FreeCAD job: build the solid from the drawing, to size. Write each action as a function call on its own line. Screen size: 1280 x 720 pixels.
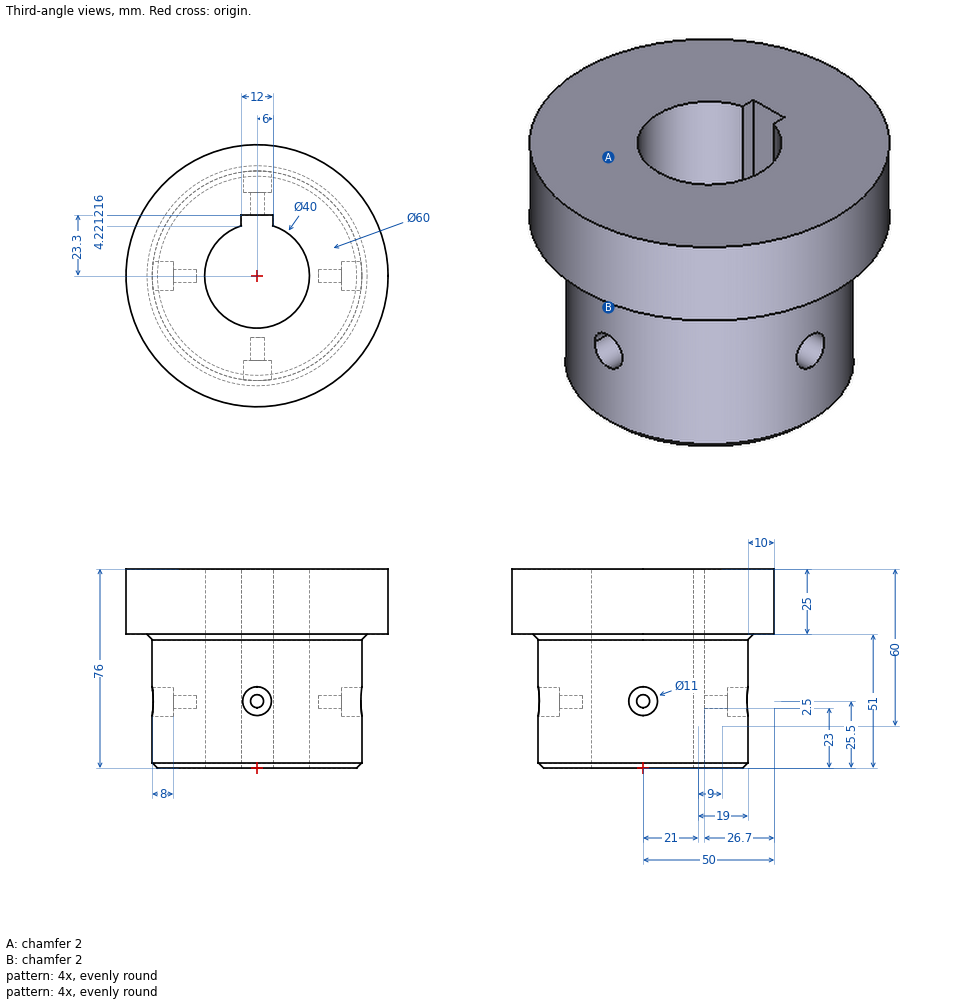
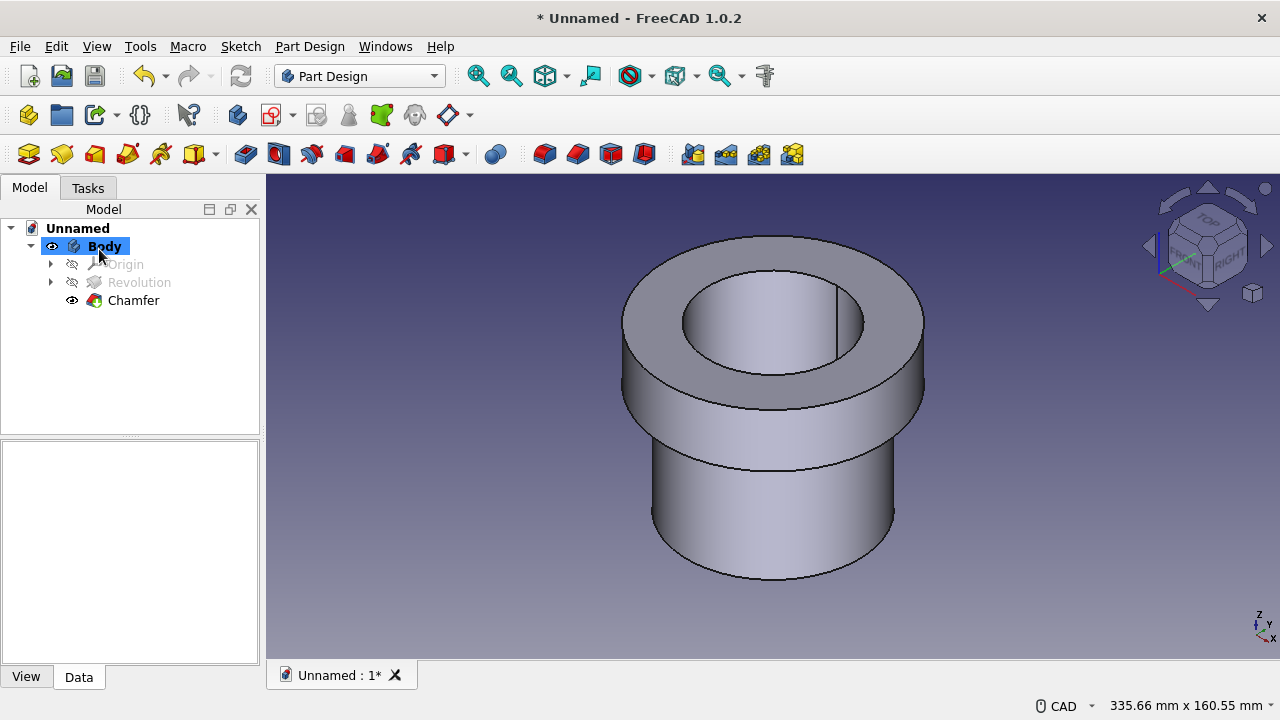
key(2)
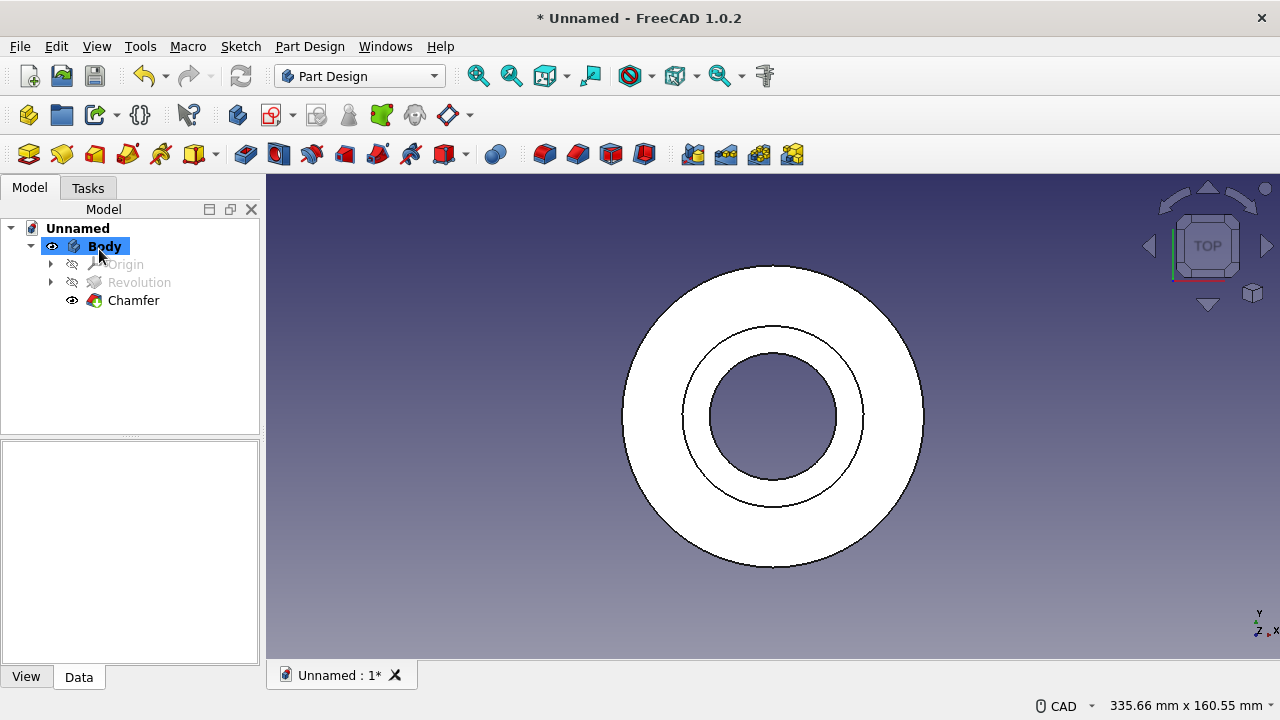
key(0)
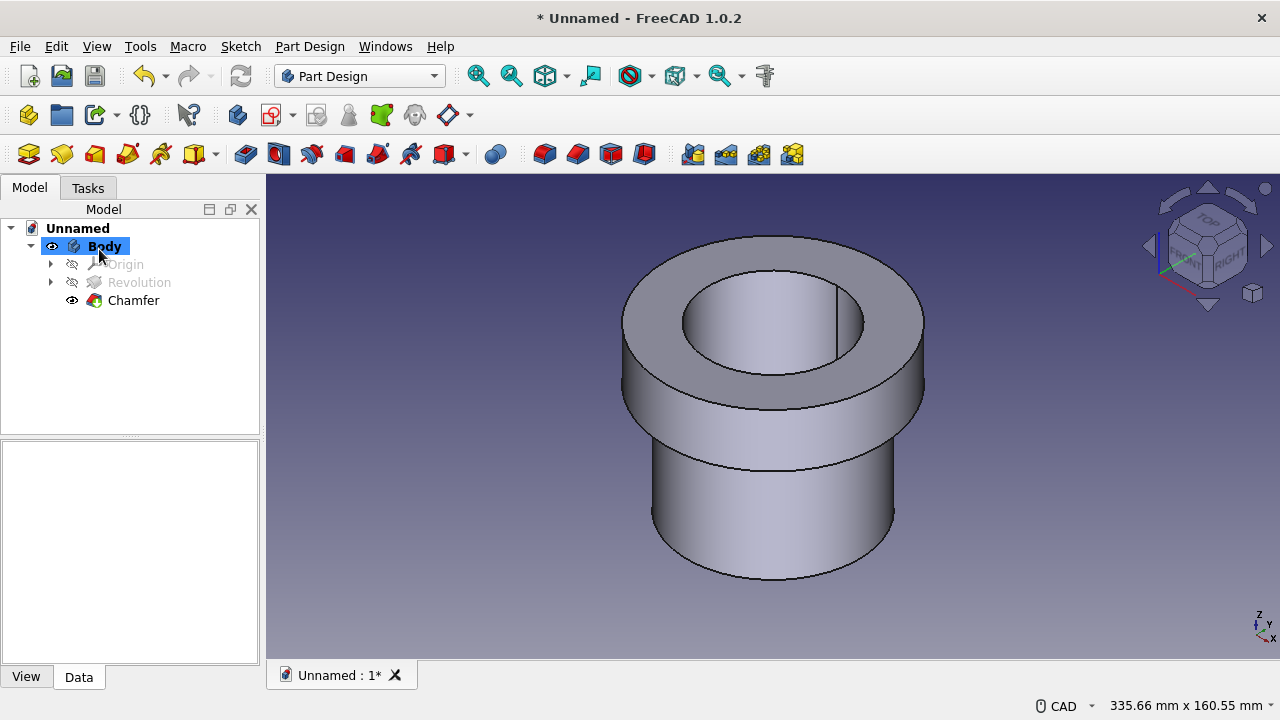
key(1)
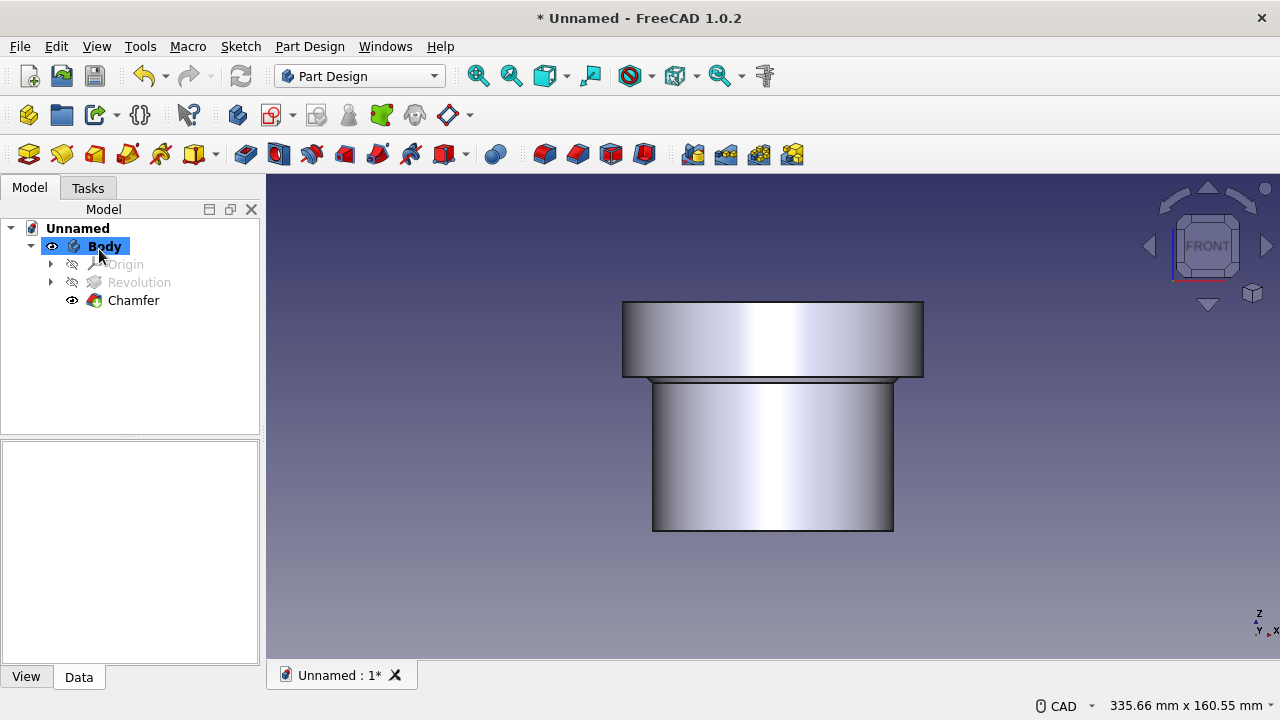
click(773, 530)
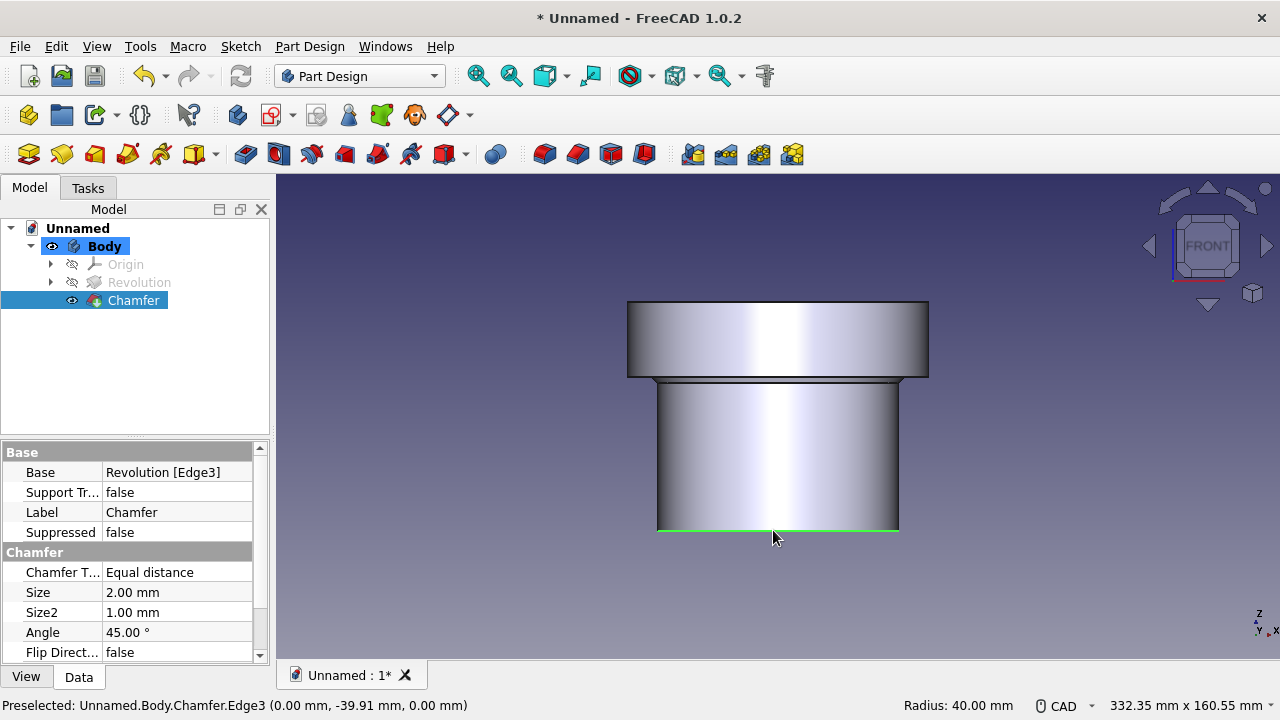
click(578, 154)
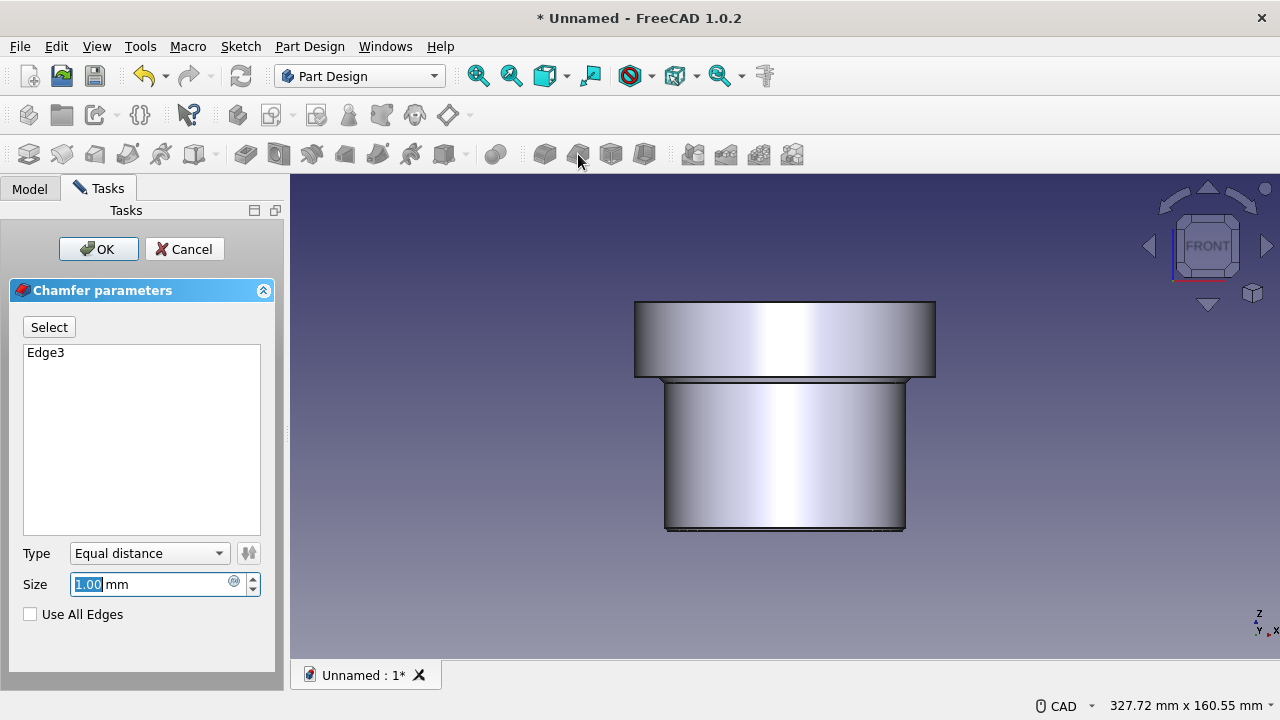
text(2)
key(Tab)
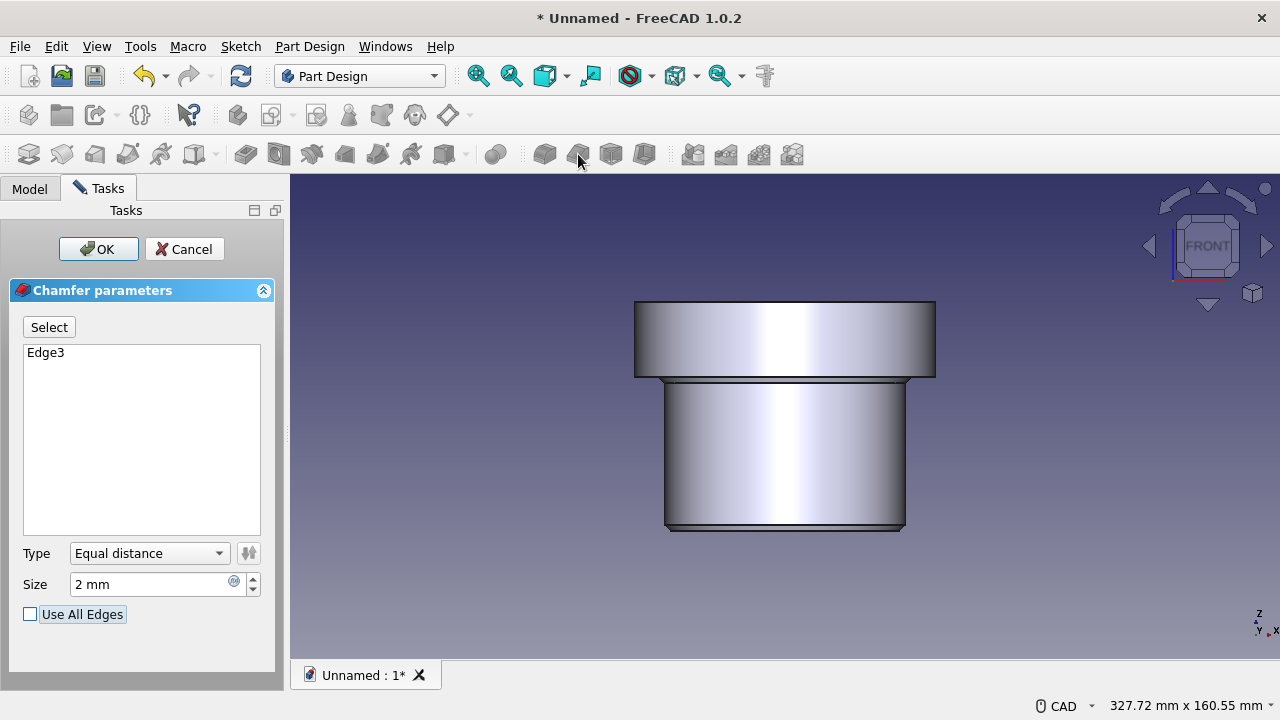
click(99, 249)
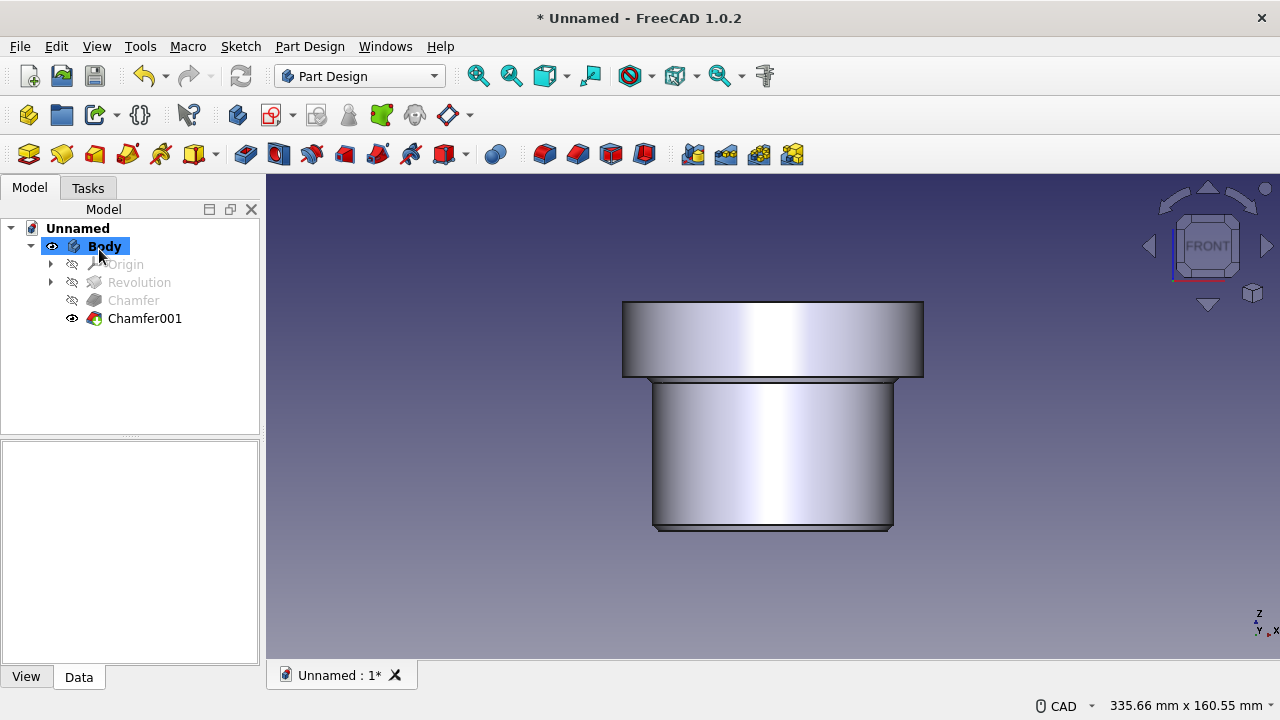
key(0)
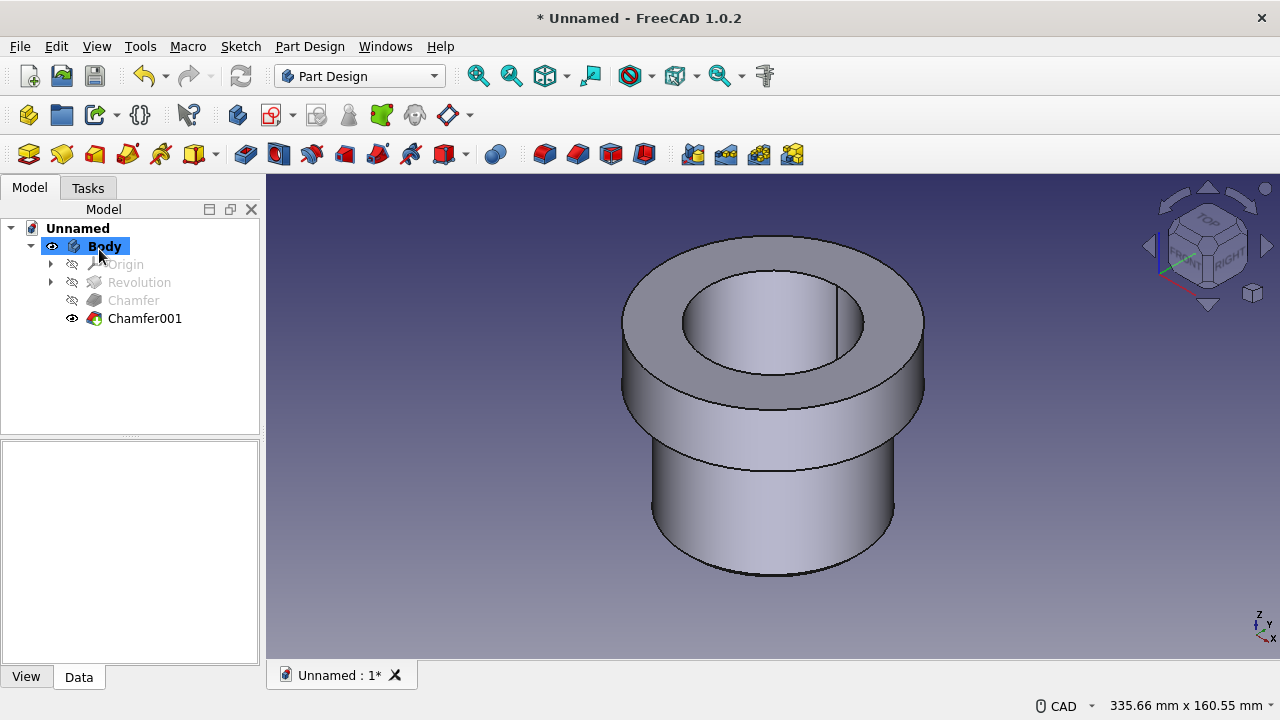
click(895, 322)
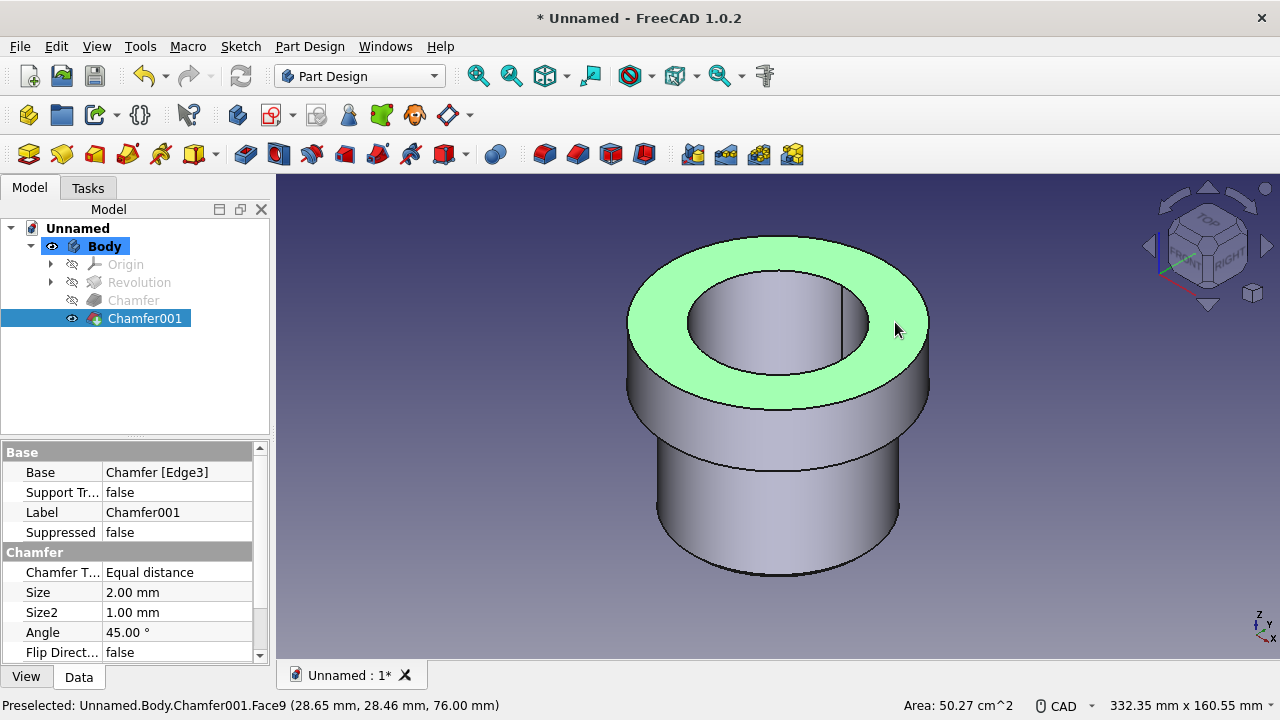
click(270, 116)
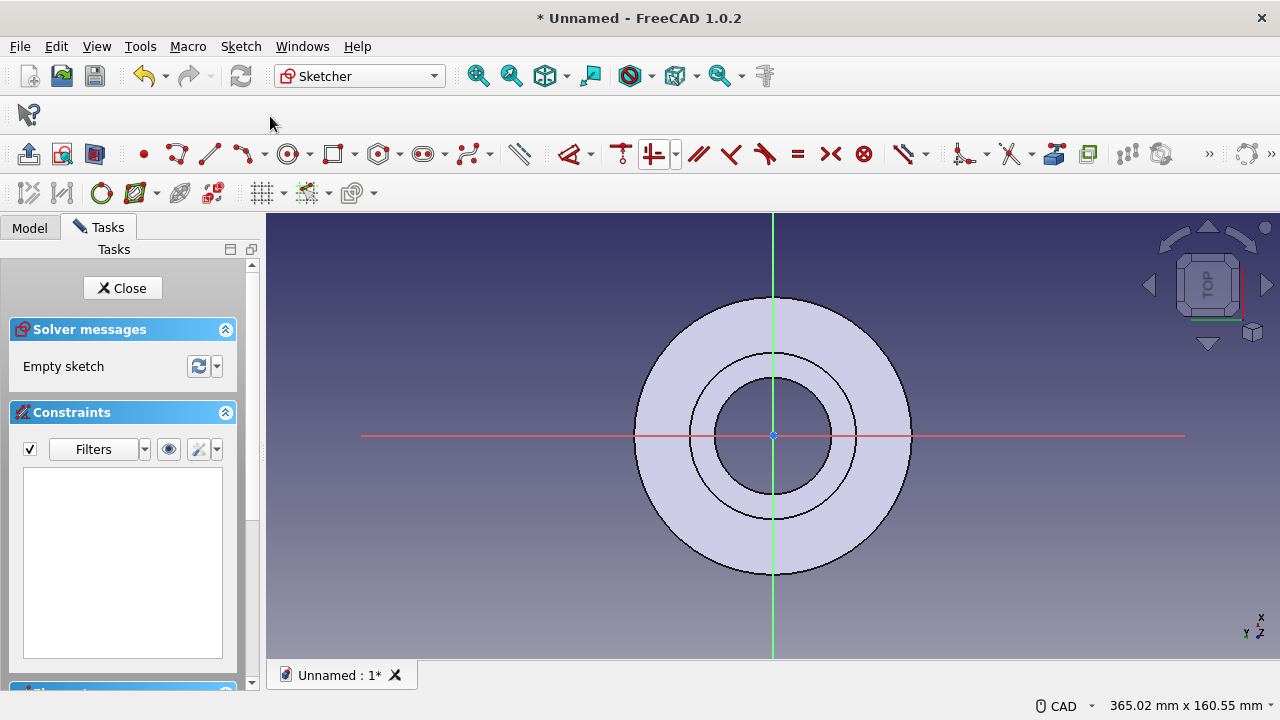
scroll(856, 436, up, 3)